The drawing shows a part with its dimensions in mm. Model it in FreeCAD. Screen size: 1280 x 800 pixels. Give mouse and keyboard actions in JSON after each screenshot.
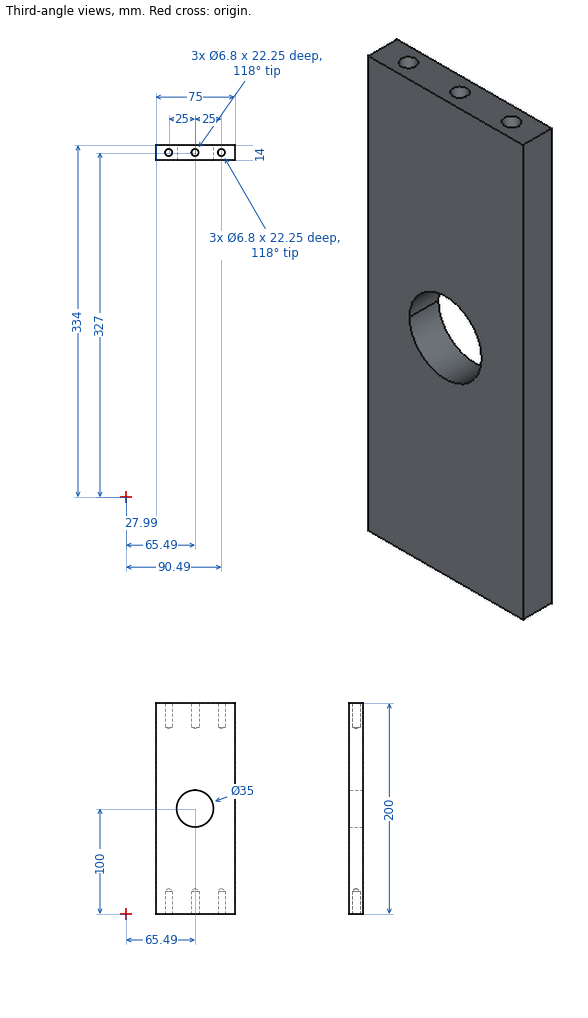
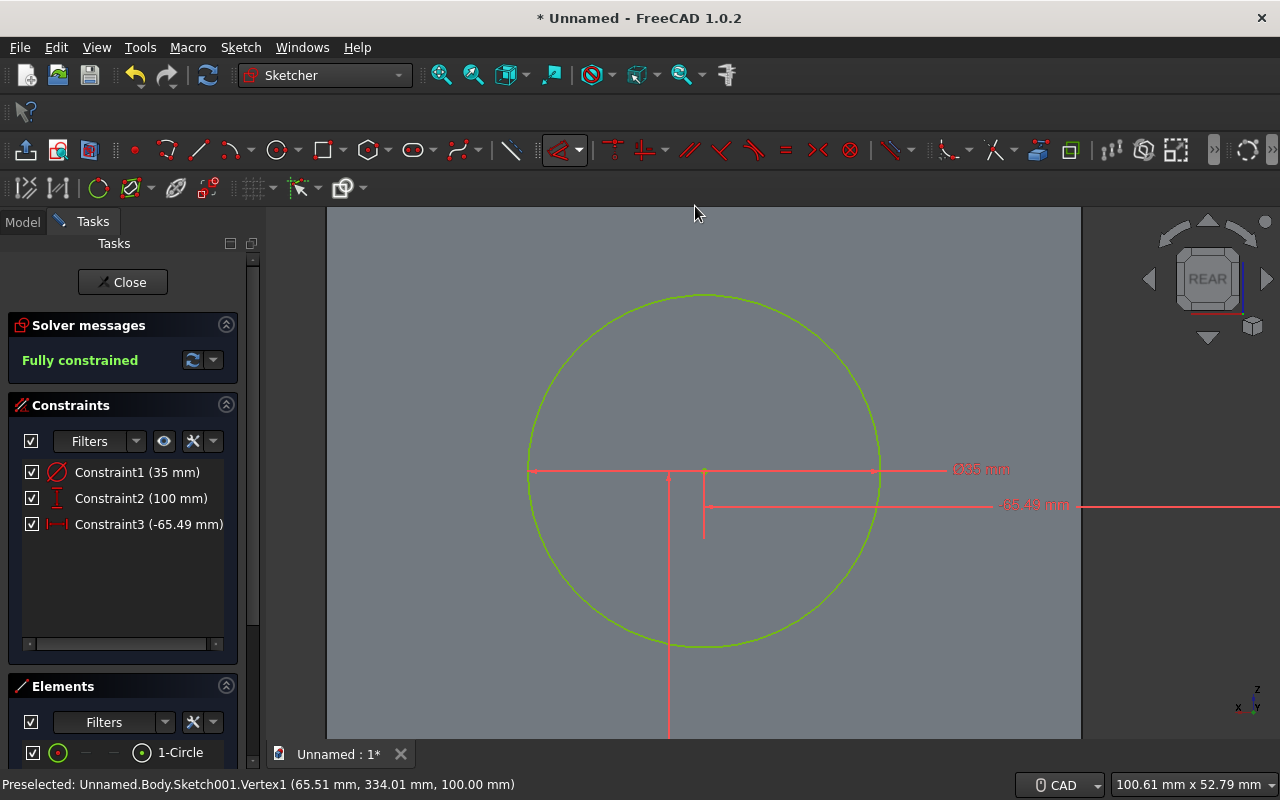
{"action": "left_click", "coordinate": [123, 282]}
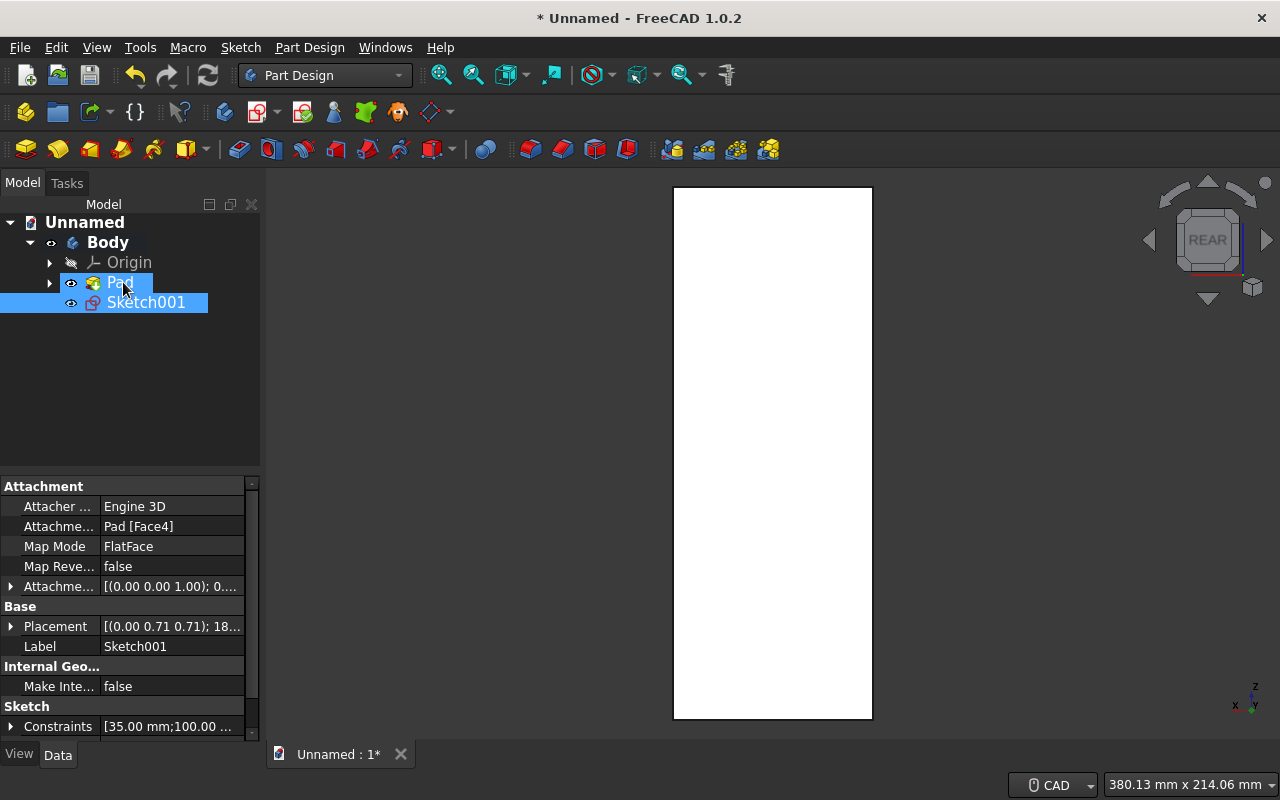
{"action": "left_click", "coordinate": [240, 150]}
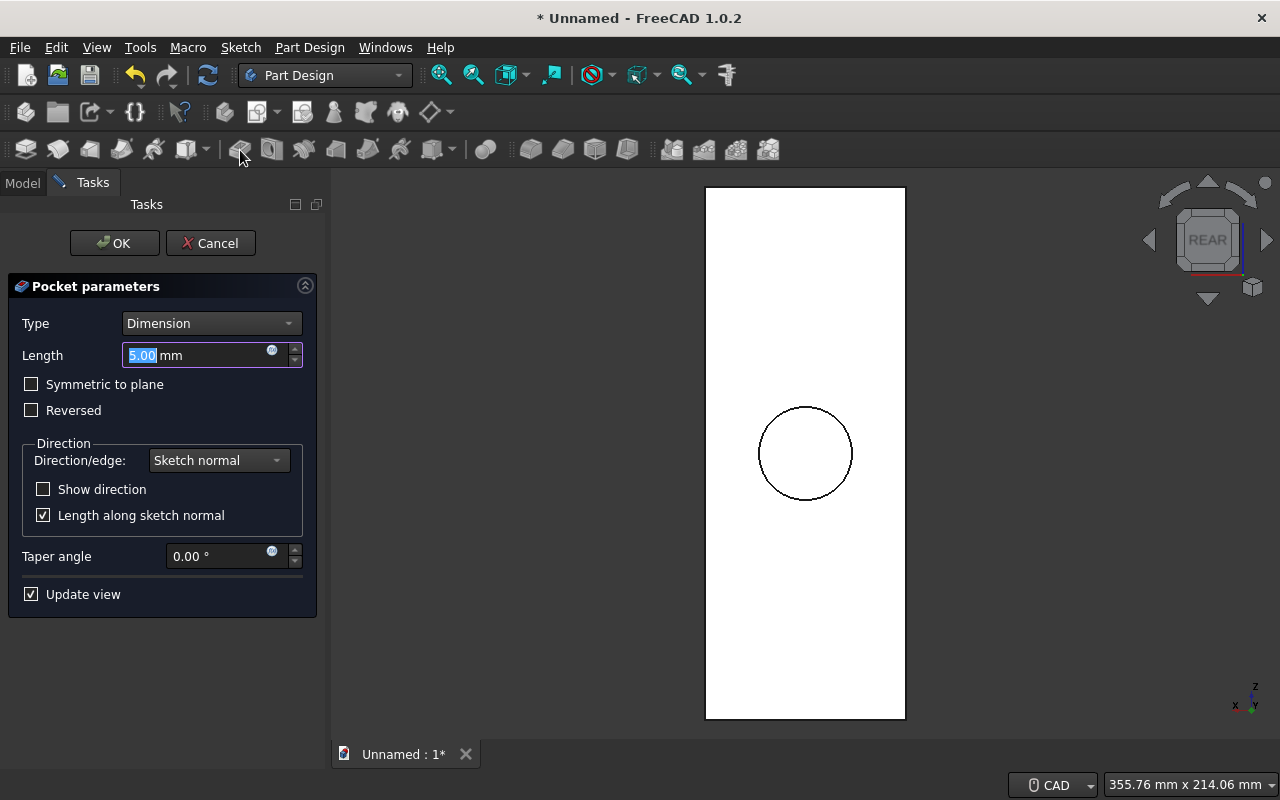
{"action": "left_click", "coordinate": [212, 324]}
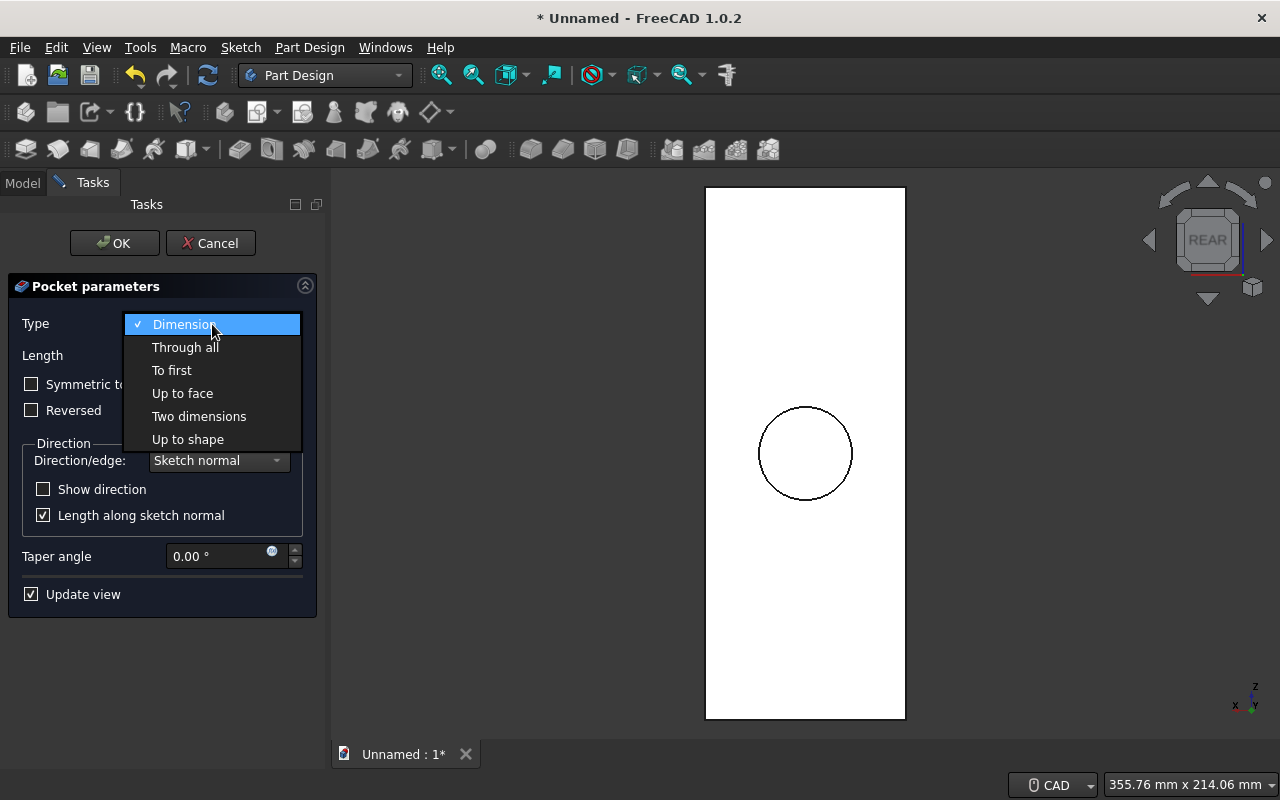
{"action": "left_click", "coordinate": [212, 348]}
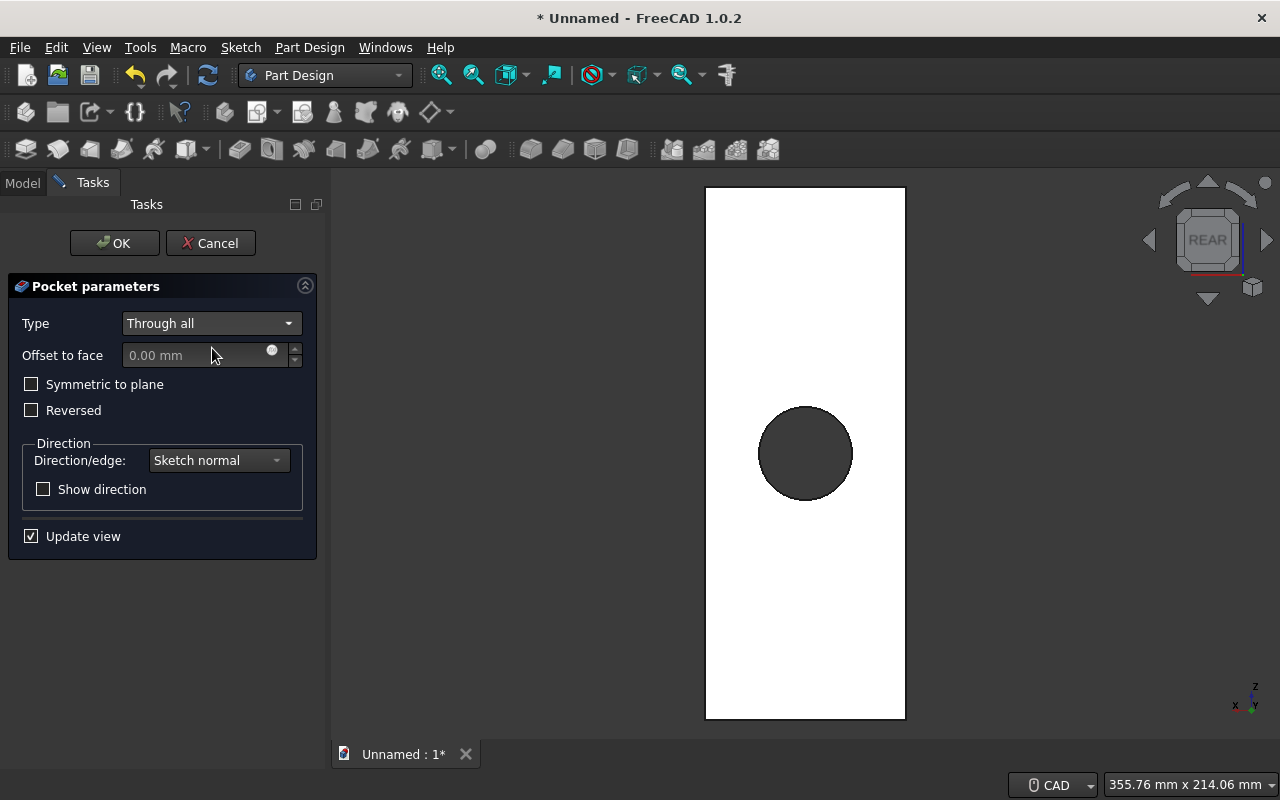
{"action": "left_click", "coordinate": [115, 243]}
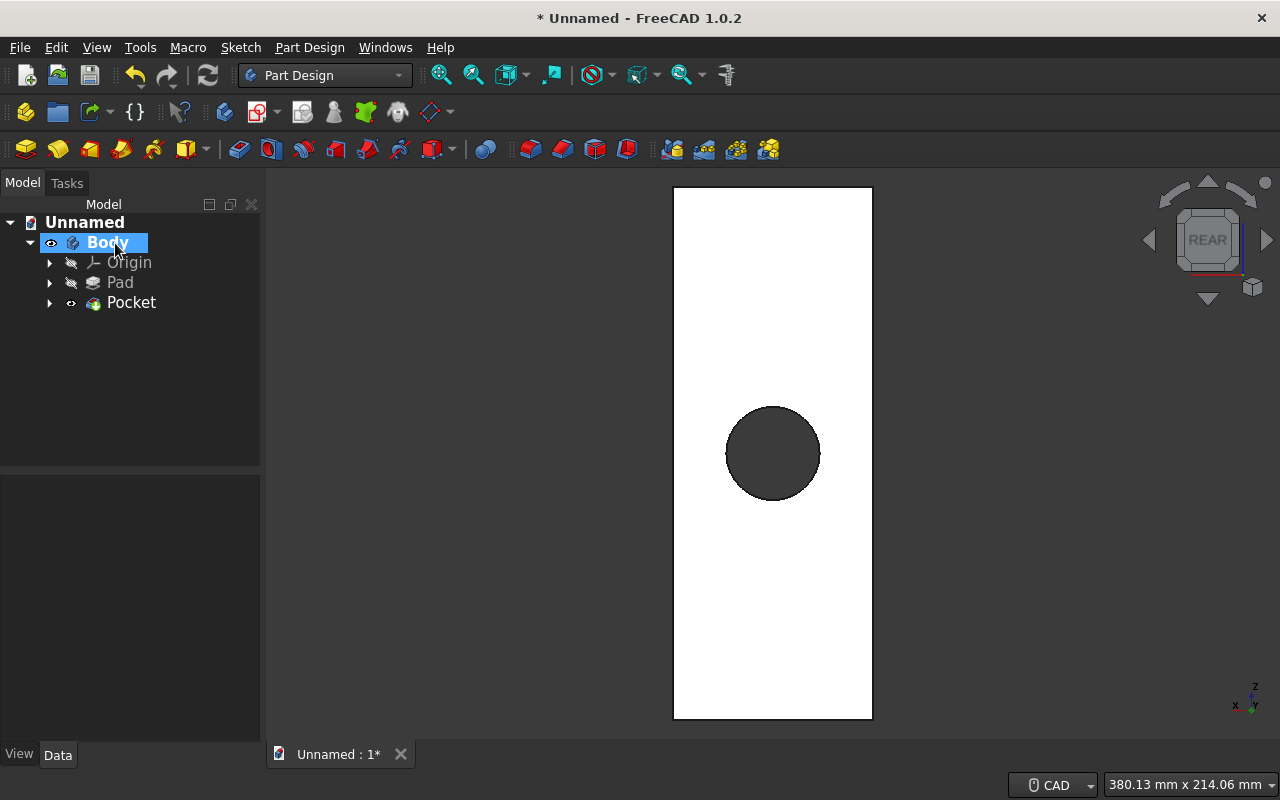
{"action": "key", "text": "0"}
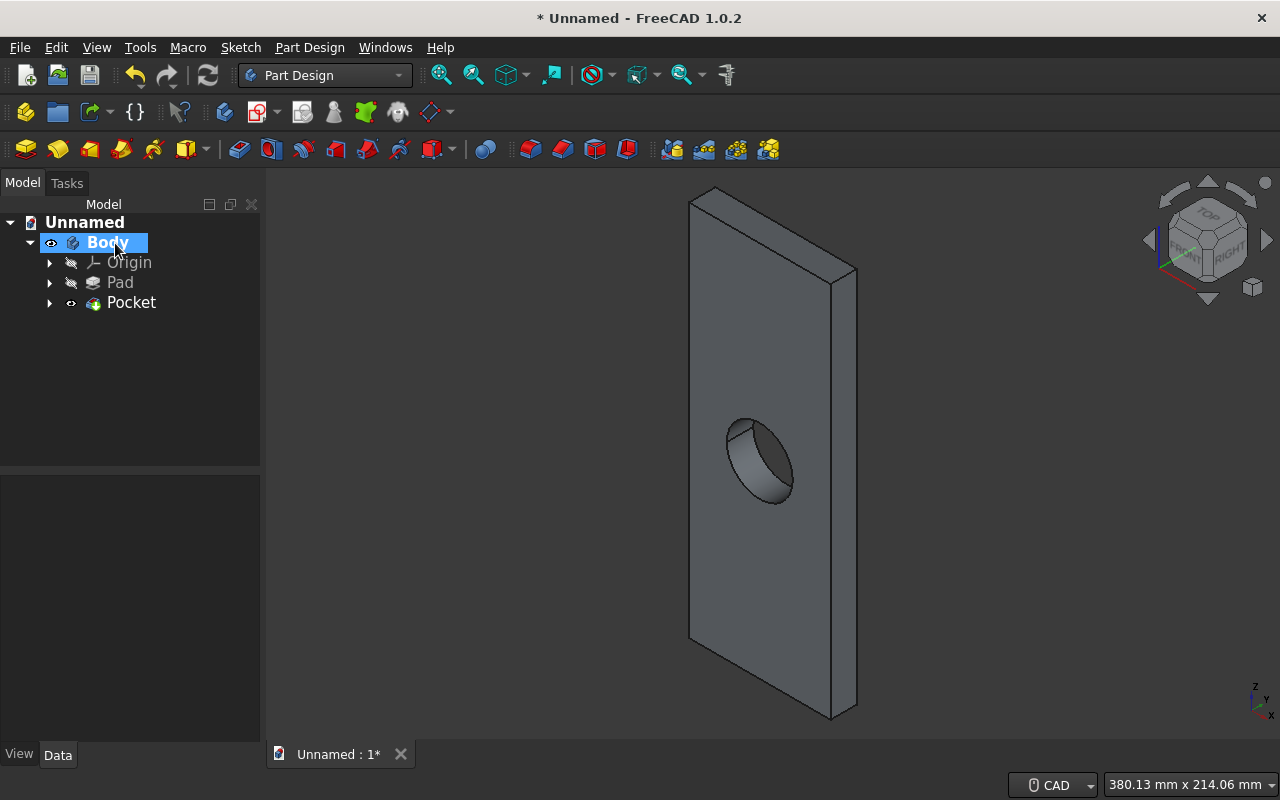
{"action": "left_click", "coordinate": [813, 258]}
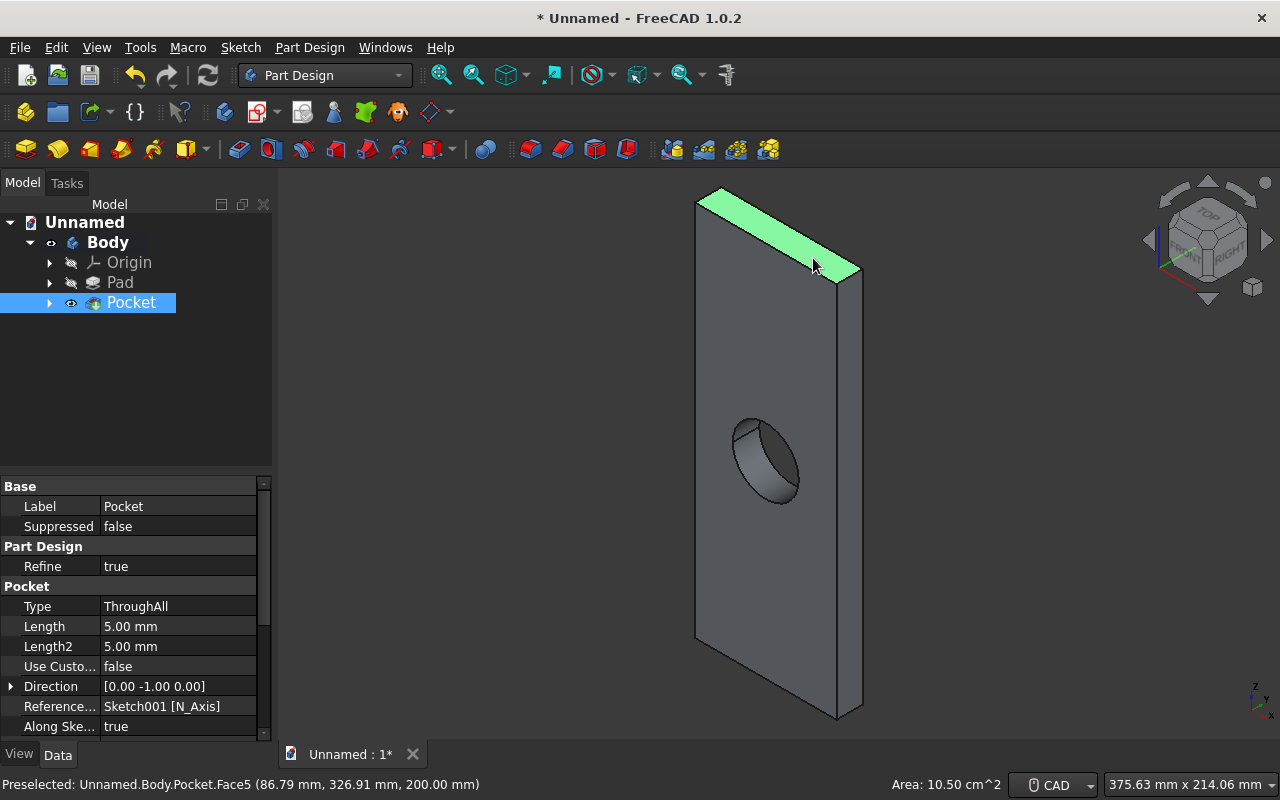
{"action": "left_click", "coordinate": [258, 112]}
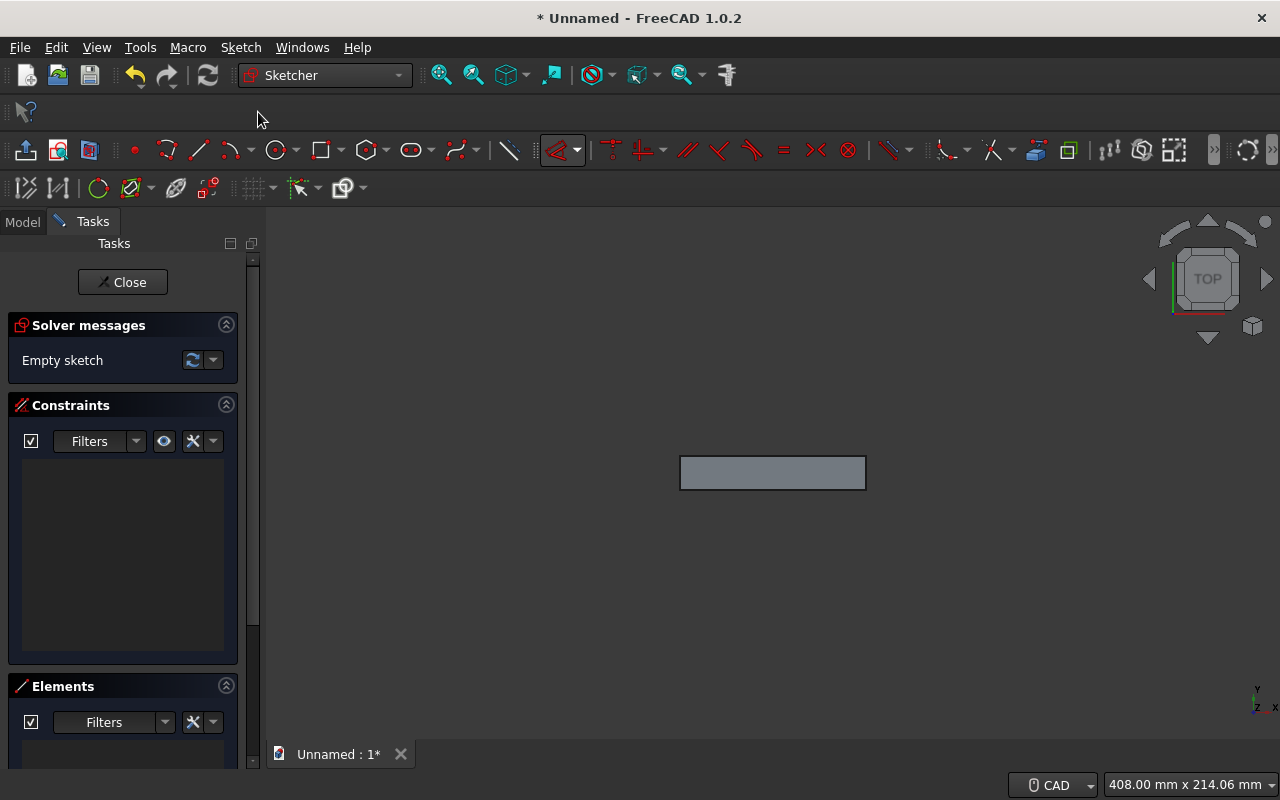
{"action": "scroll", "coordinate": [795, 473], "scroll_direction": "up", "scroll_amount": 7}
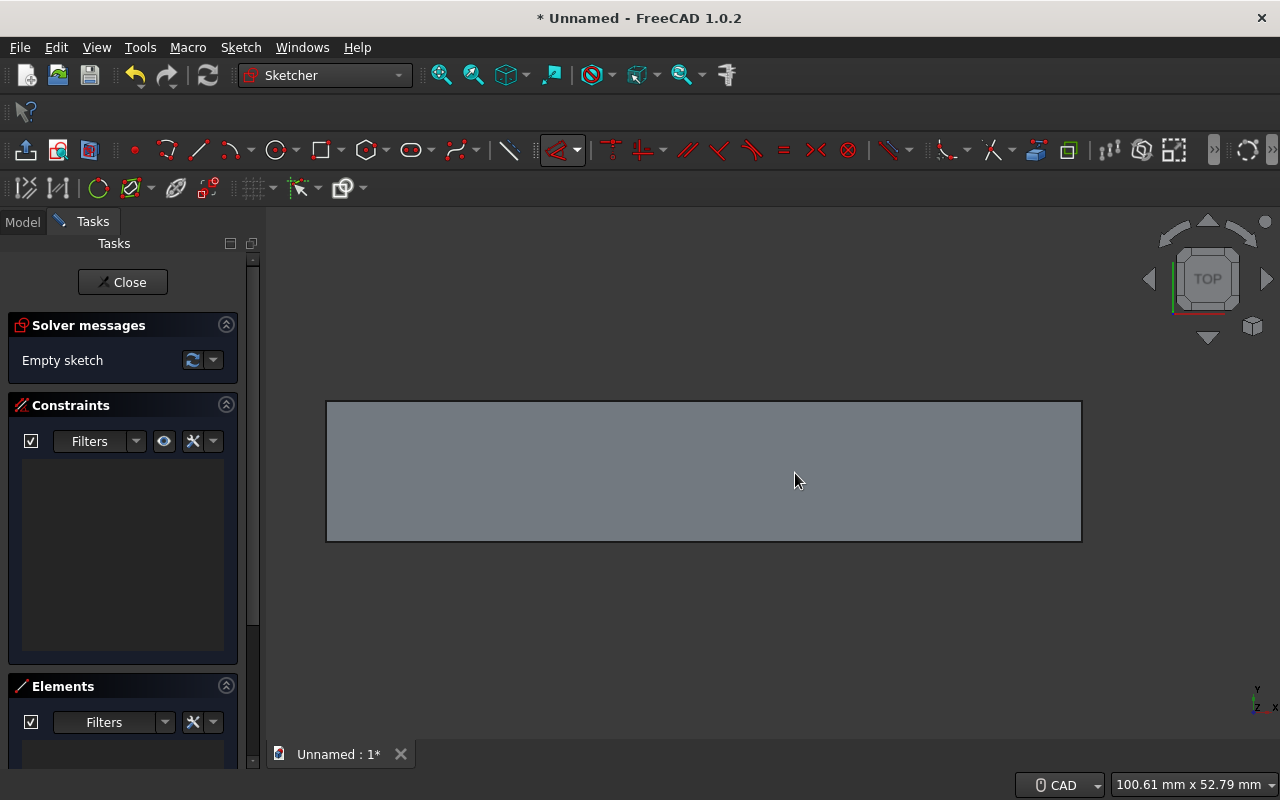
{"action": "left_click", "coordinate": [276, 150]}